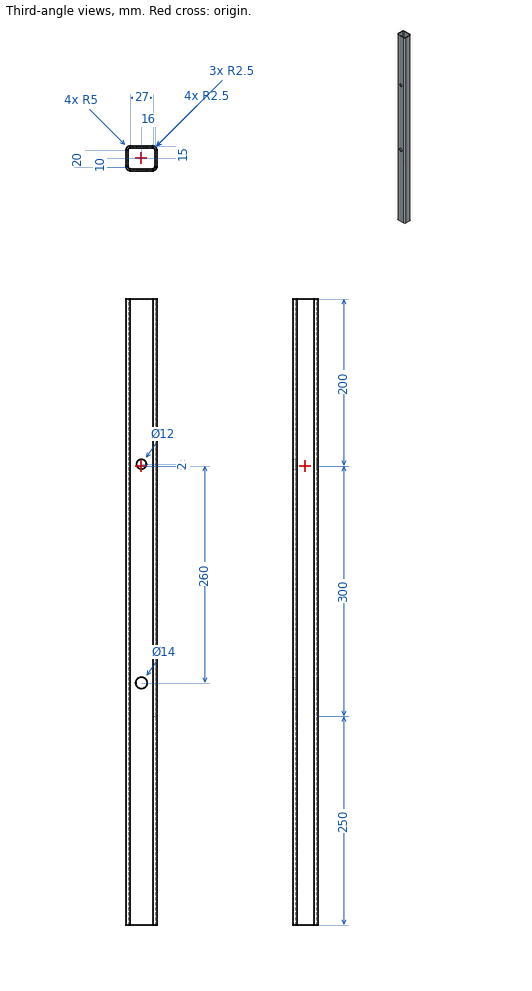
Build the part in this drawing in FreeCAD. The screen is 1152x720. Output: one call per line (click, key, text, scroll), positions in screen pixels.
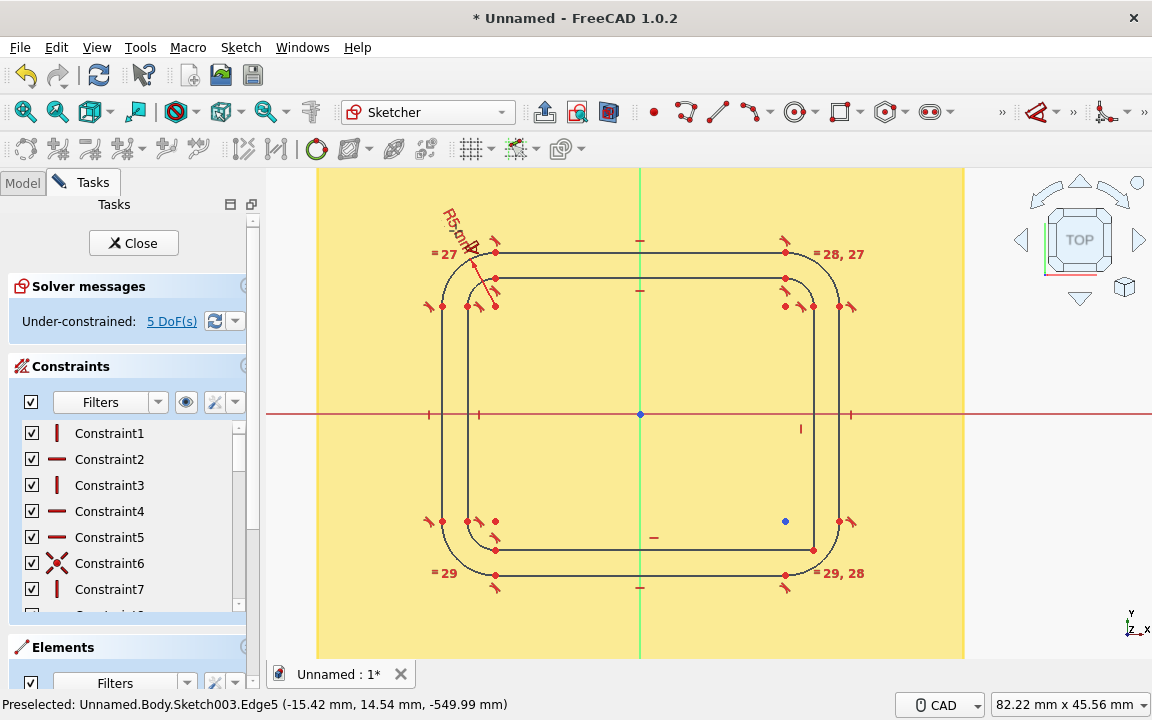
scroll(811, 294, up, 2)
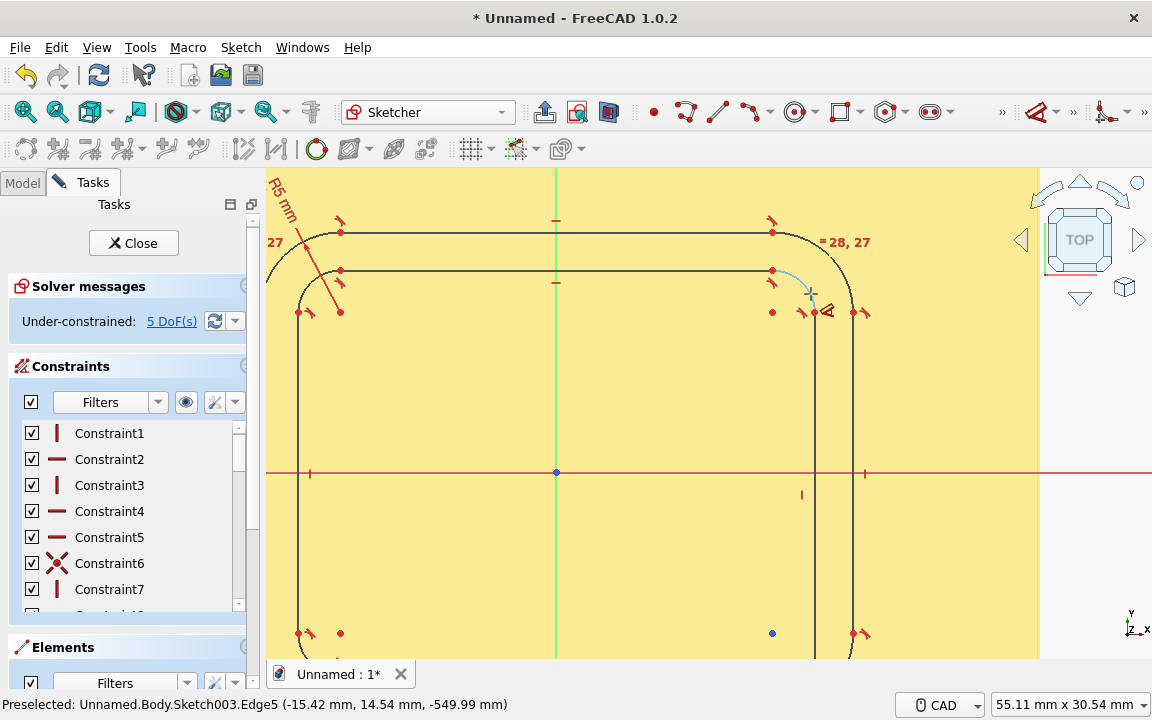
click(810, 294)
click(836, 350)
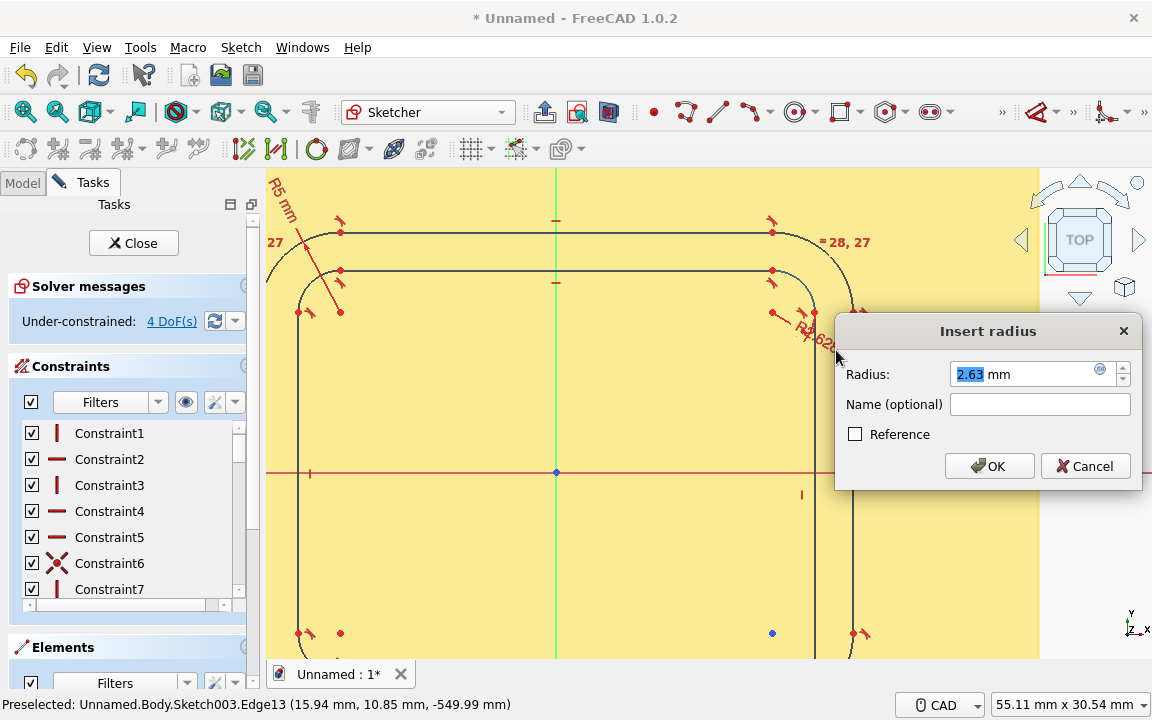
text(2.5)
key(Return)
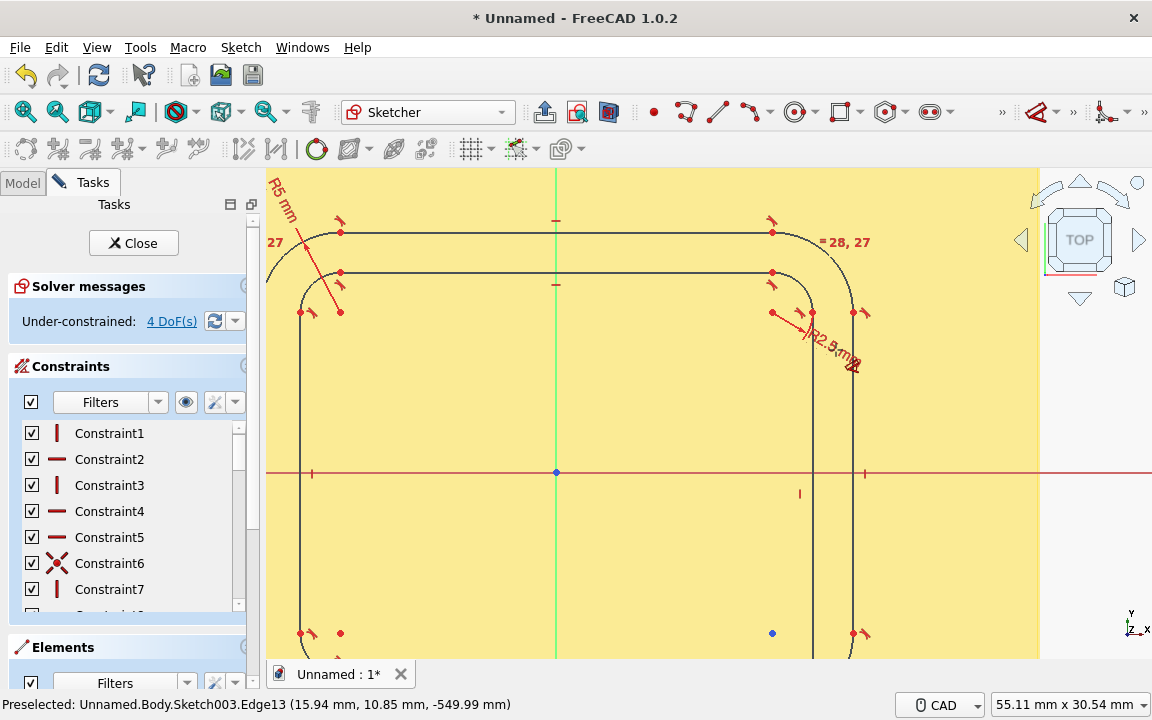
scroll(812, 293, down, 2)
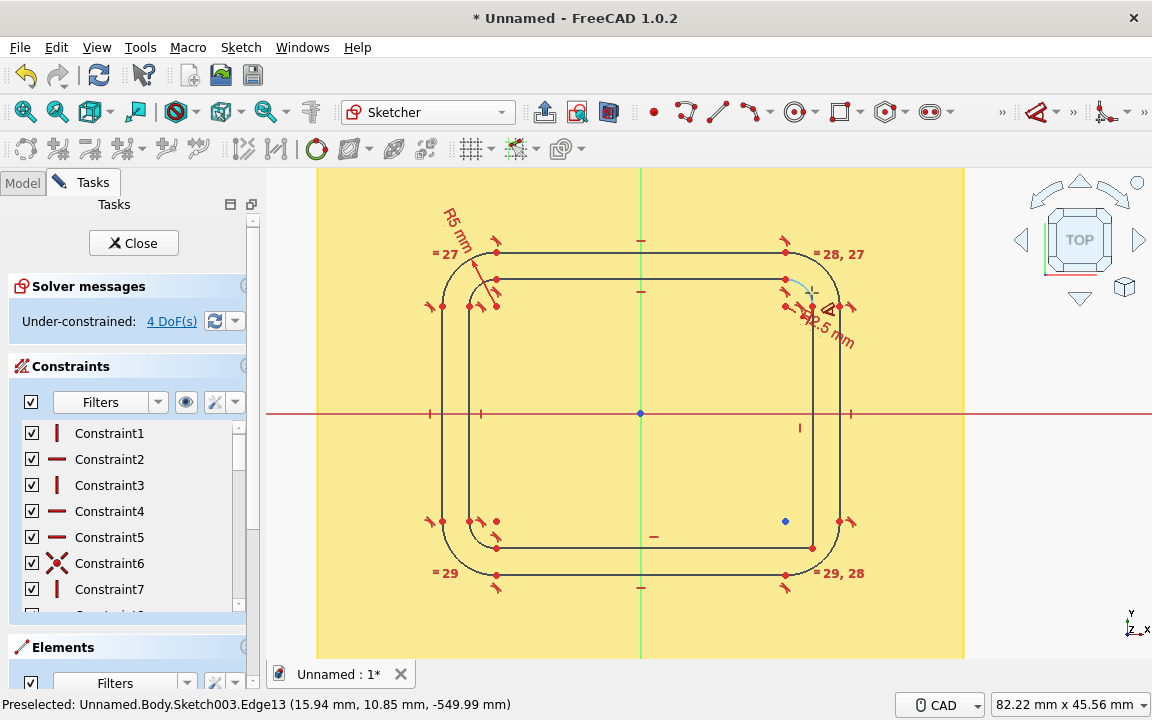
click(442, 457)
click(408, 364)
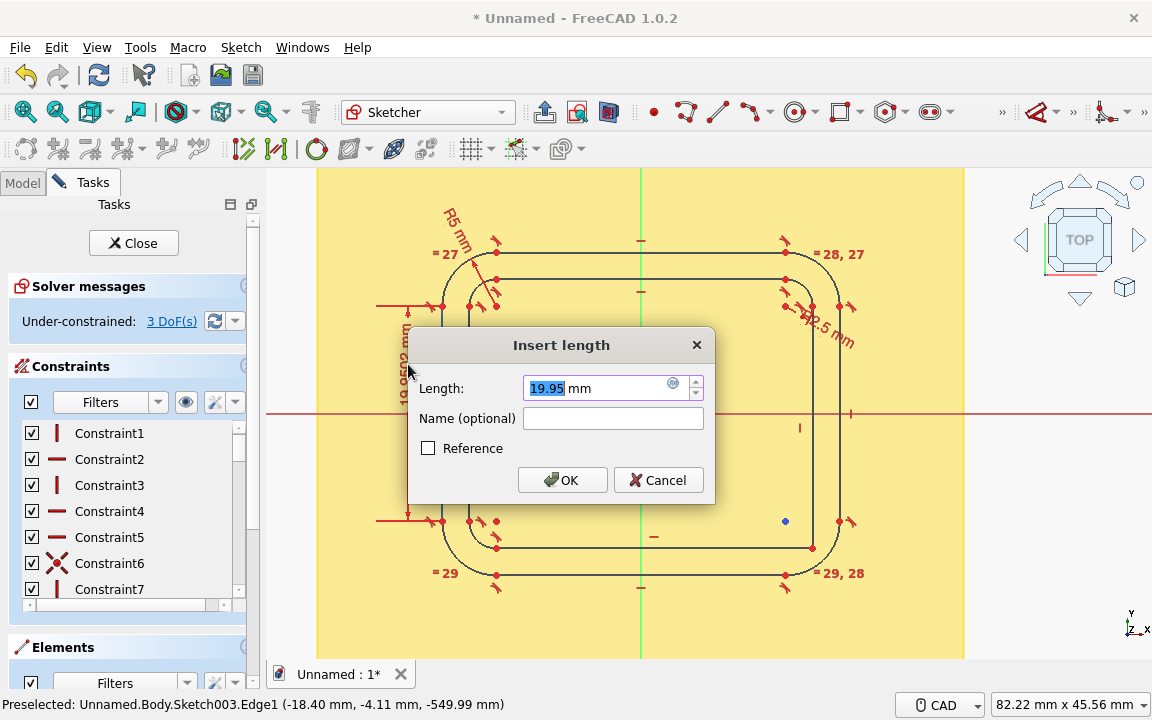
text(20)
key(Return)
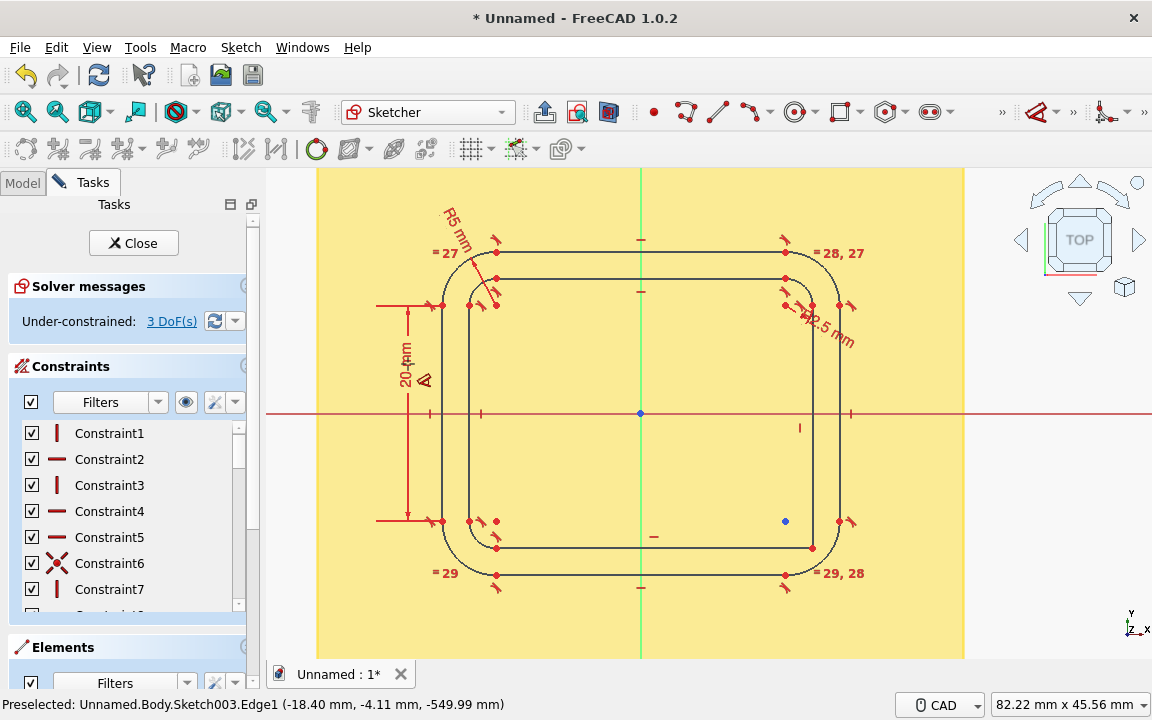
click(583, 252)
click(574, 218)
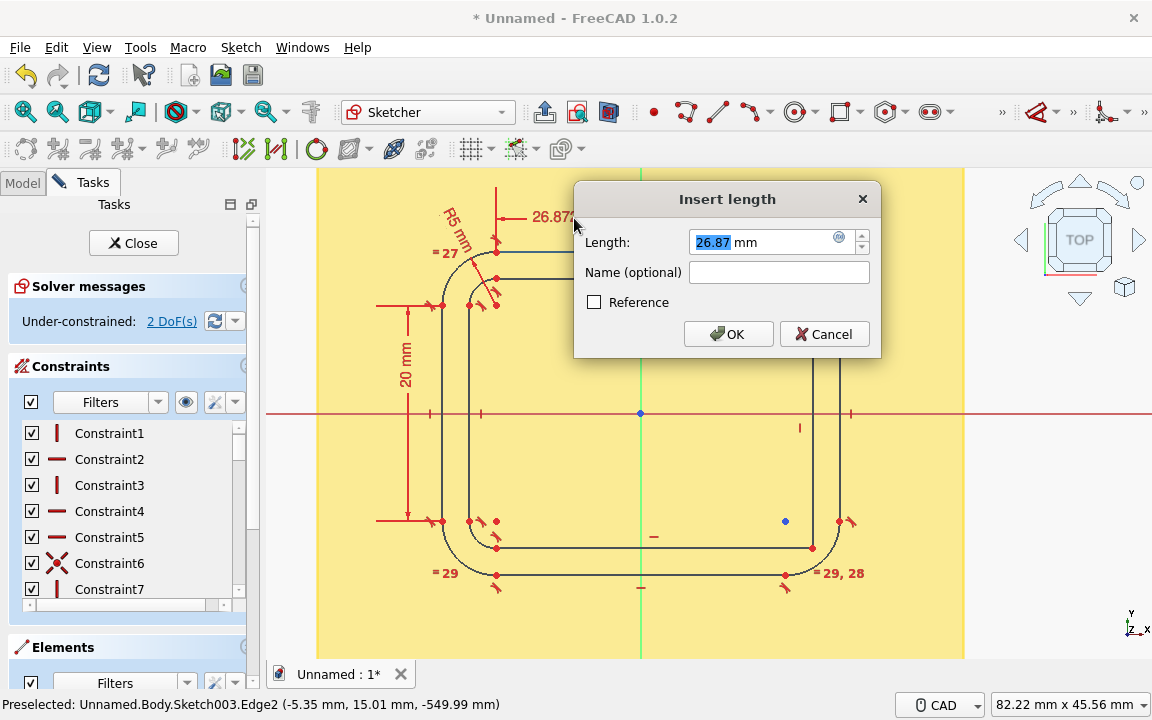
text(27)
key(Return)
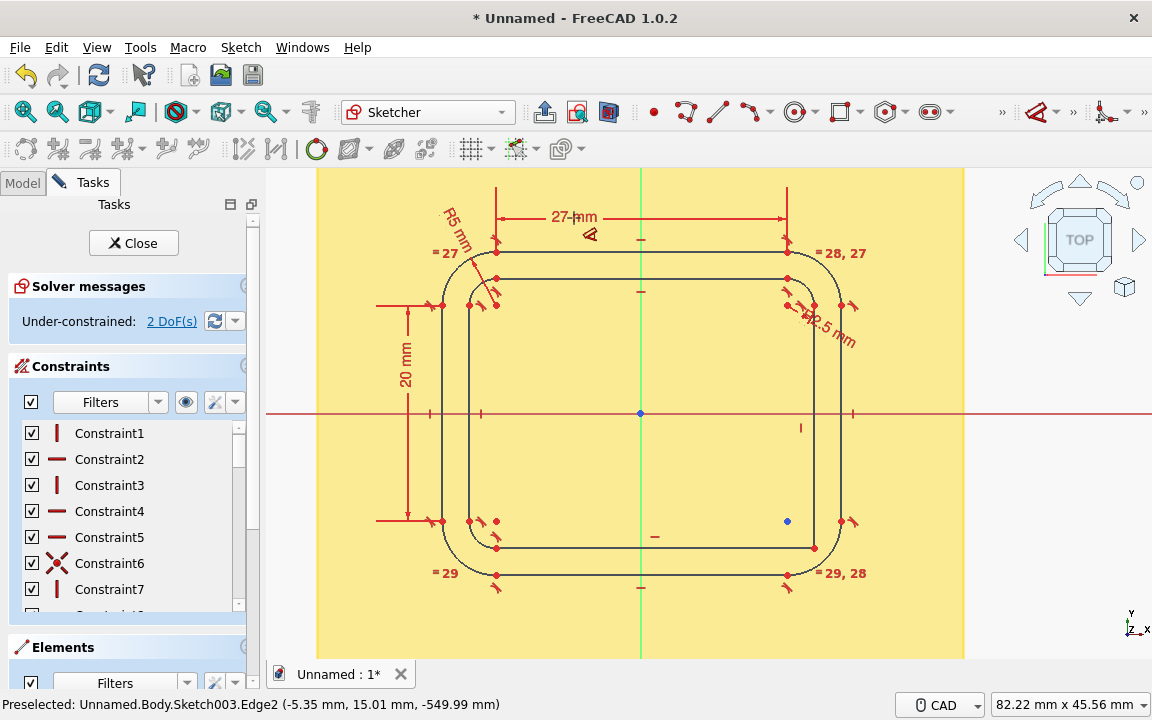
click(442, 521)
click(408, 468)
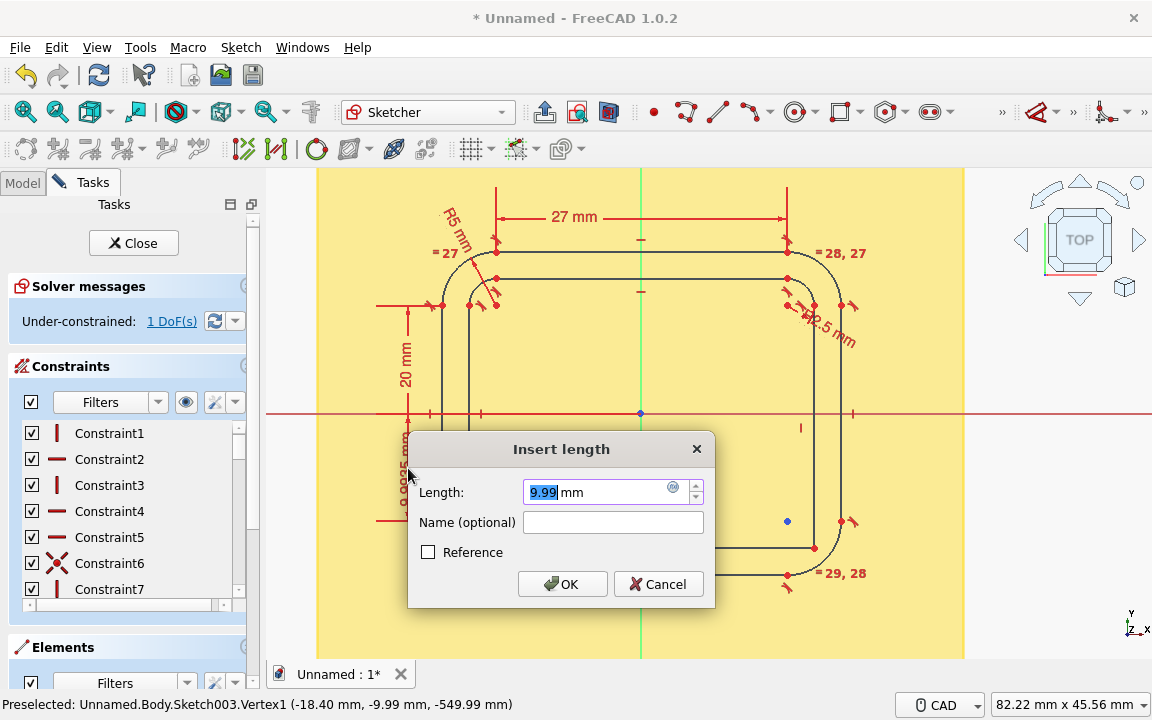
text(10)
key(Return)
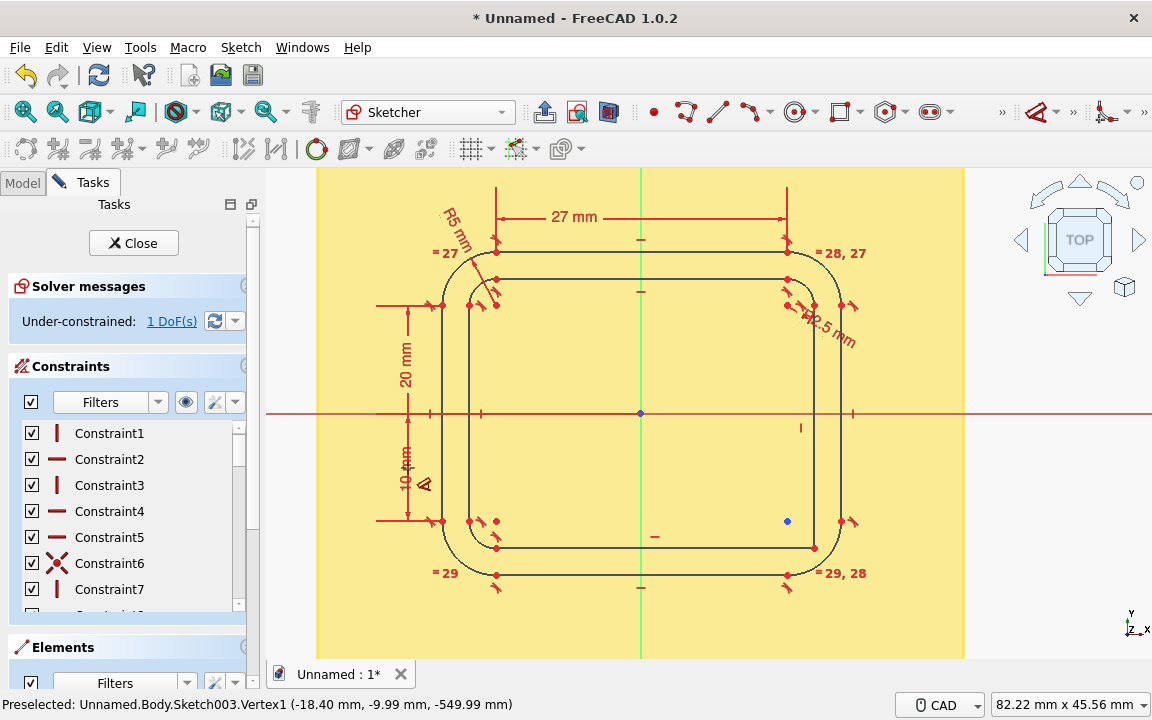
click(814, 548)
click(727, 380)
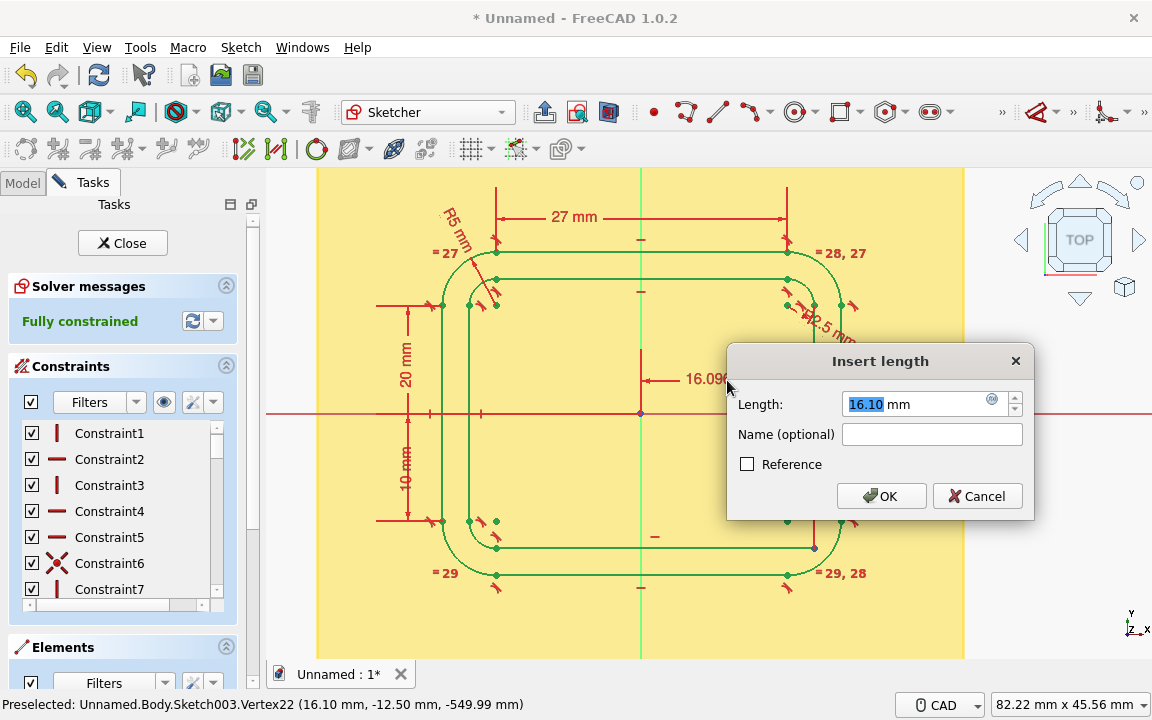
text(16)
key(Return)
key(Escape)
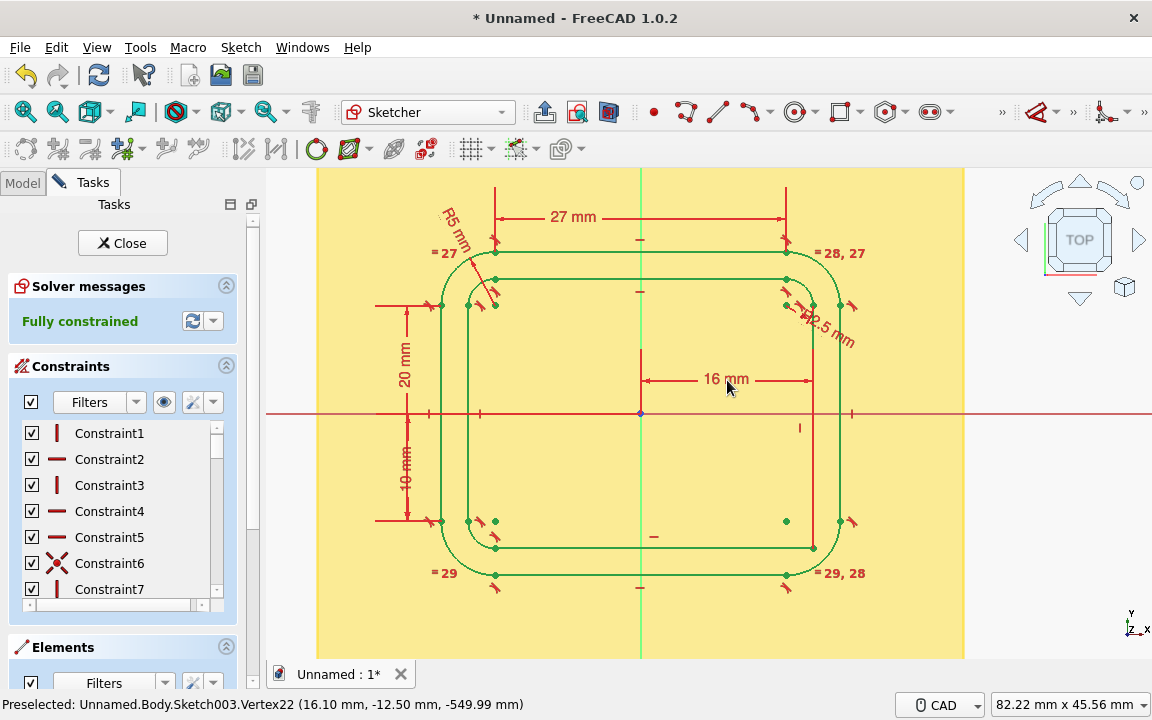
click(123, 243)